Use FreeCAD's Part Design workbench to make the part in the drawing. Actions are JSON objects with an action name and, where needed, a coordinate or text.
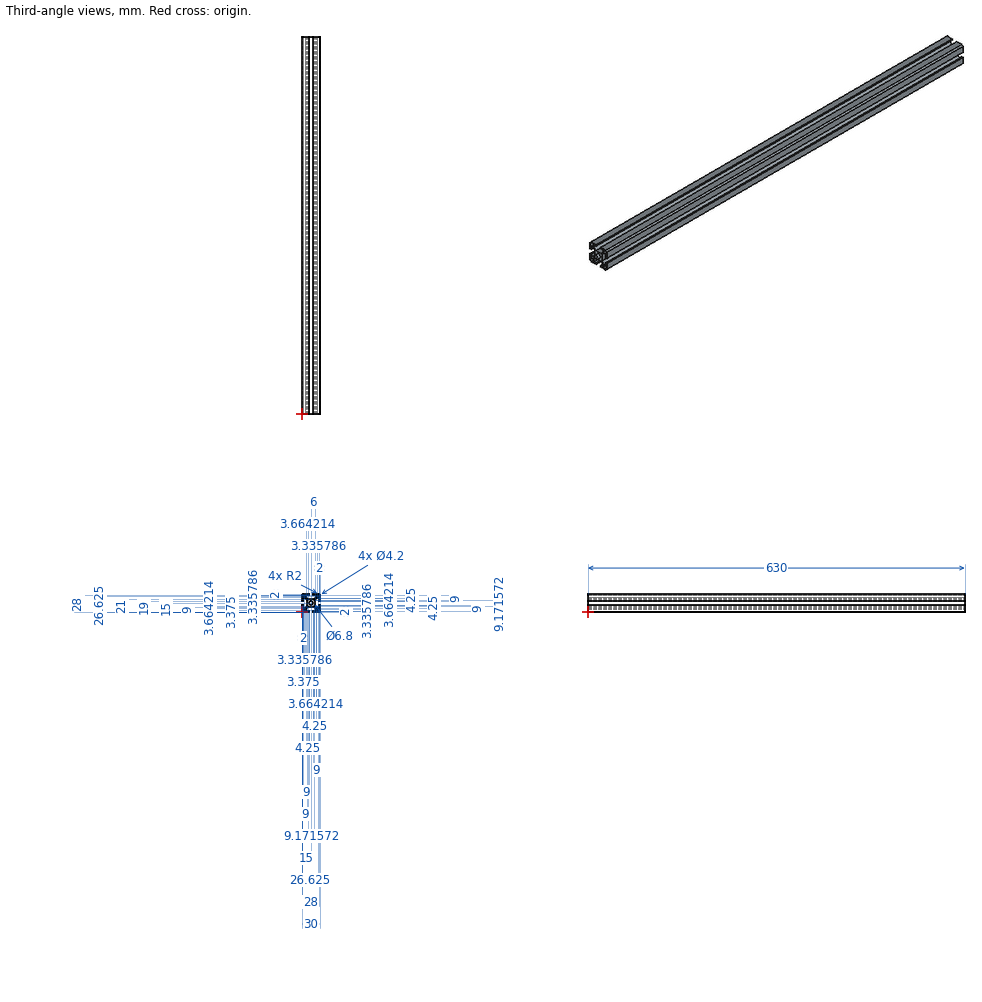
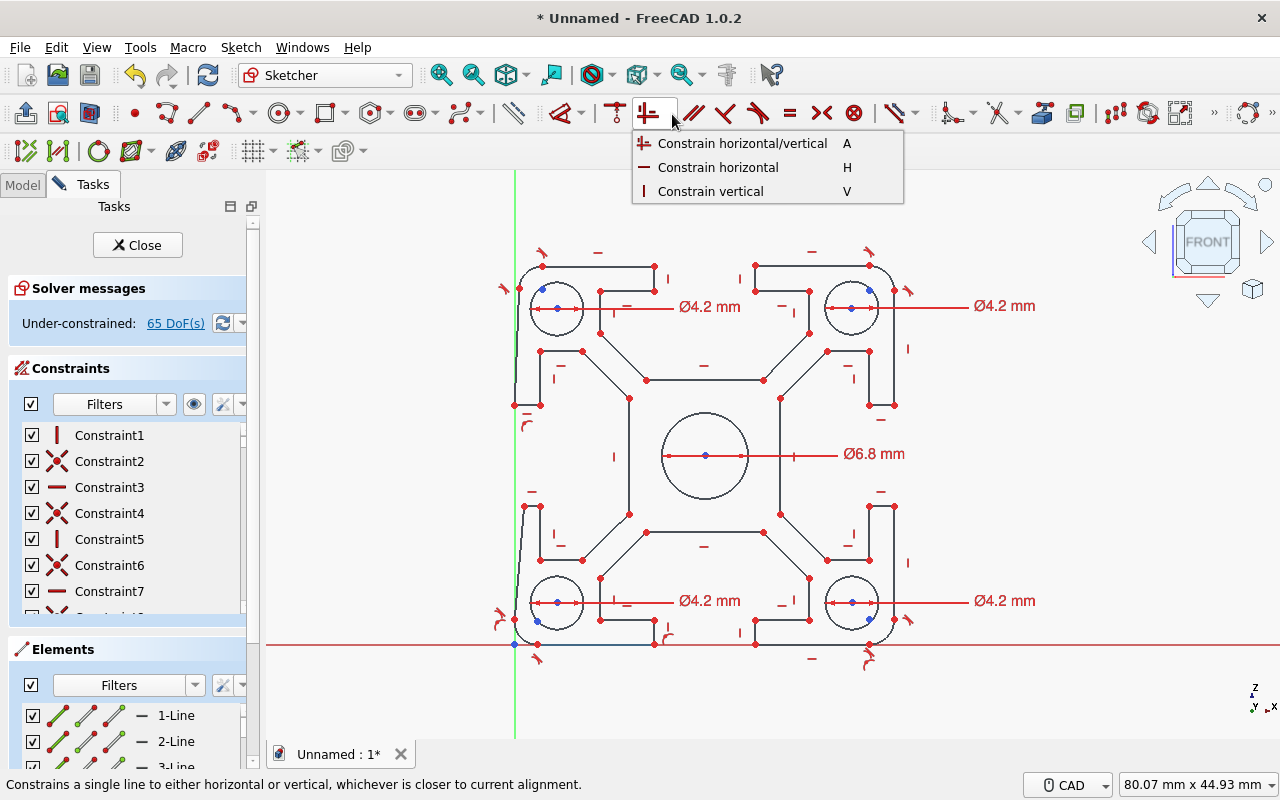
{"action": "left_click", "coordinate": [768, 167]}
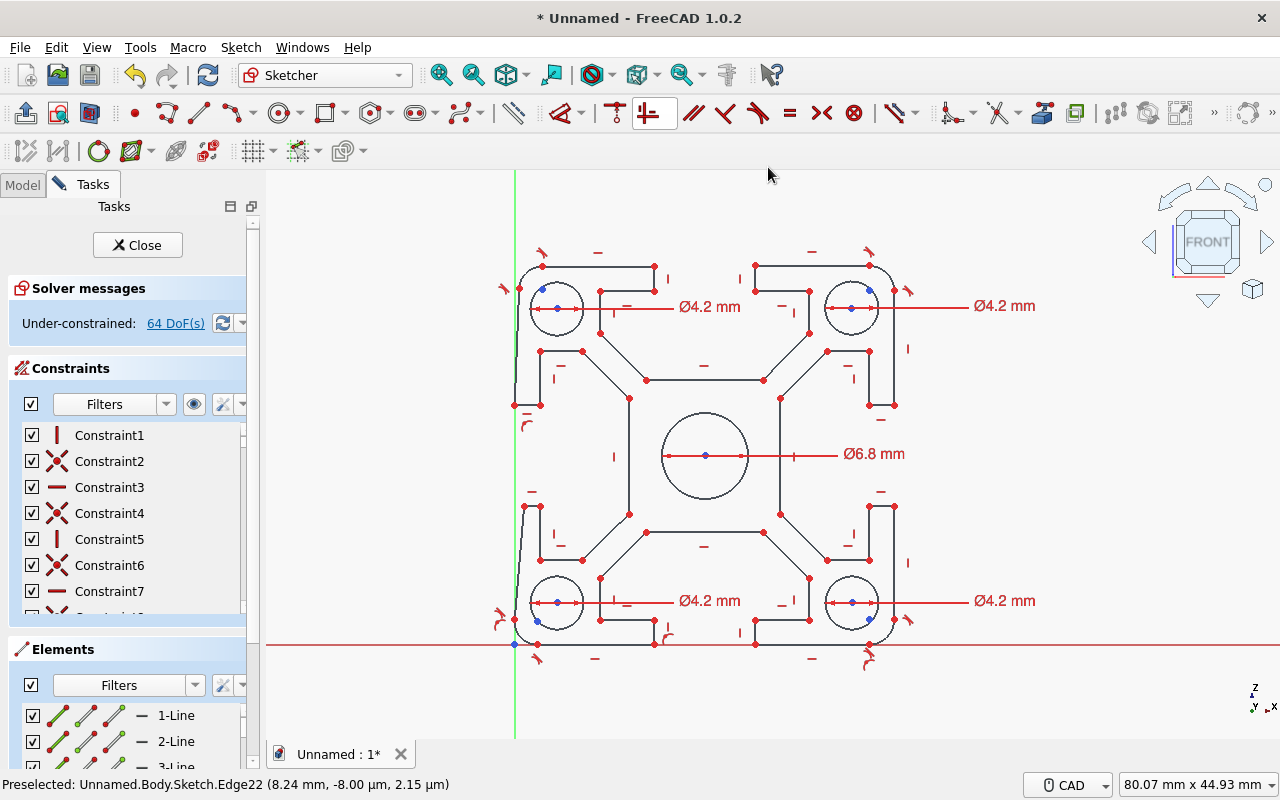
{"action": "left_click", "coordinate": [517, 586]}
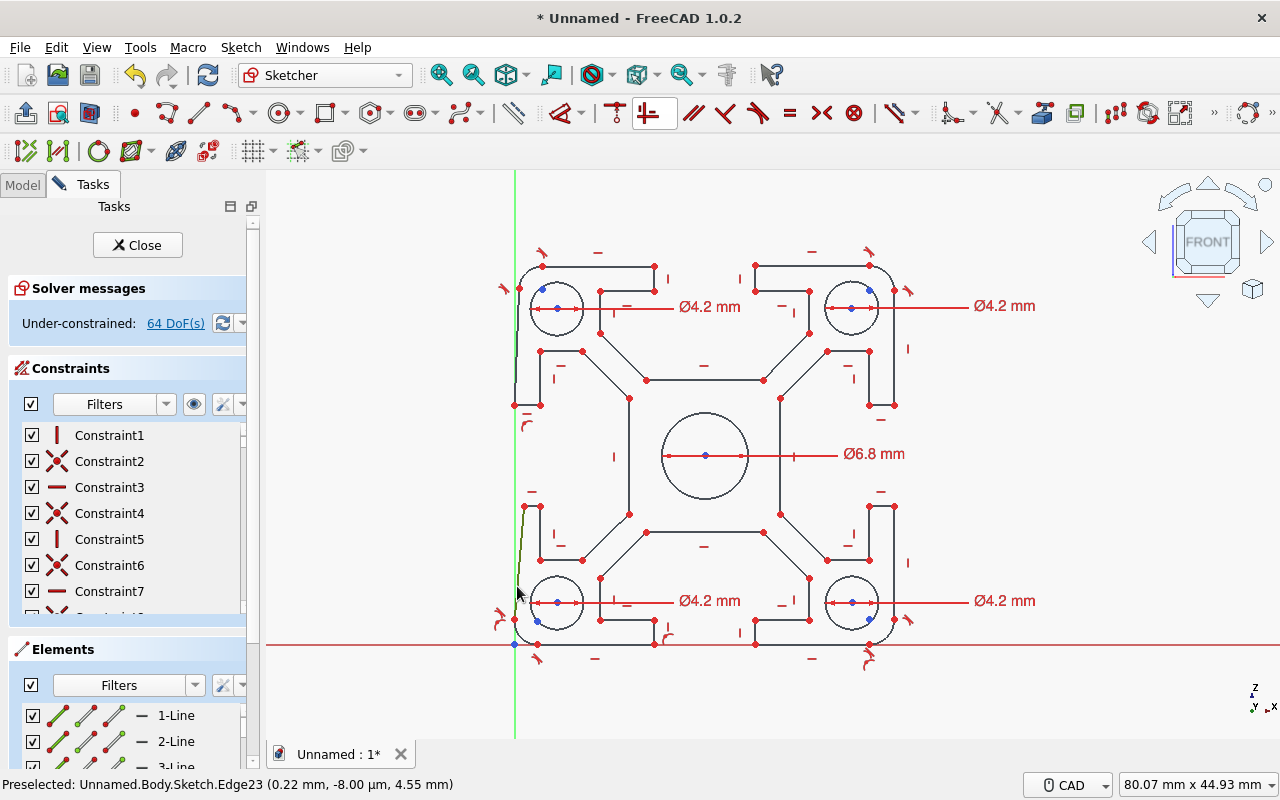
{"action": "left_click", "coordinate": [672, 114]}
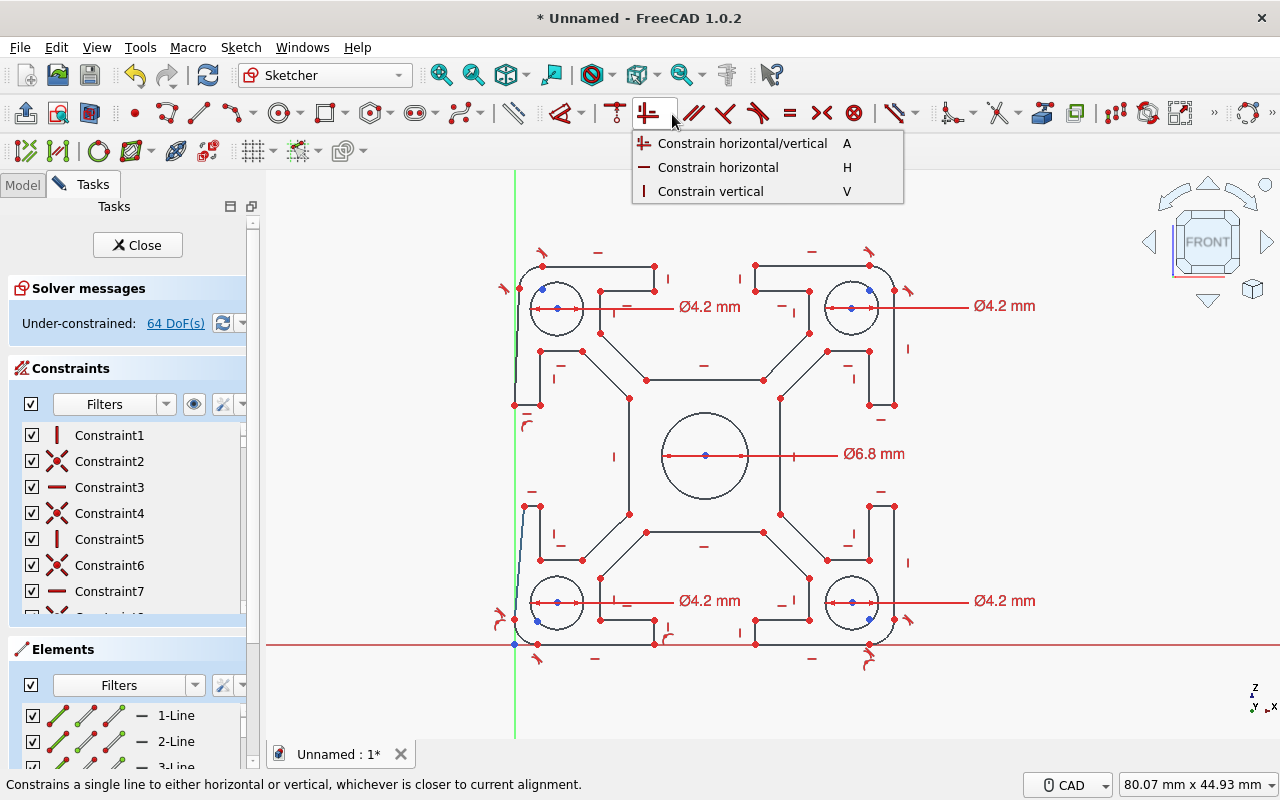
{"action": "left_click", "coordinate": [768, 191]}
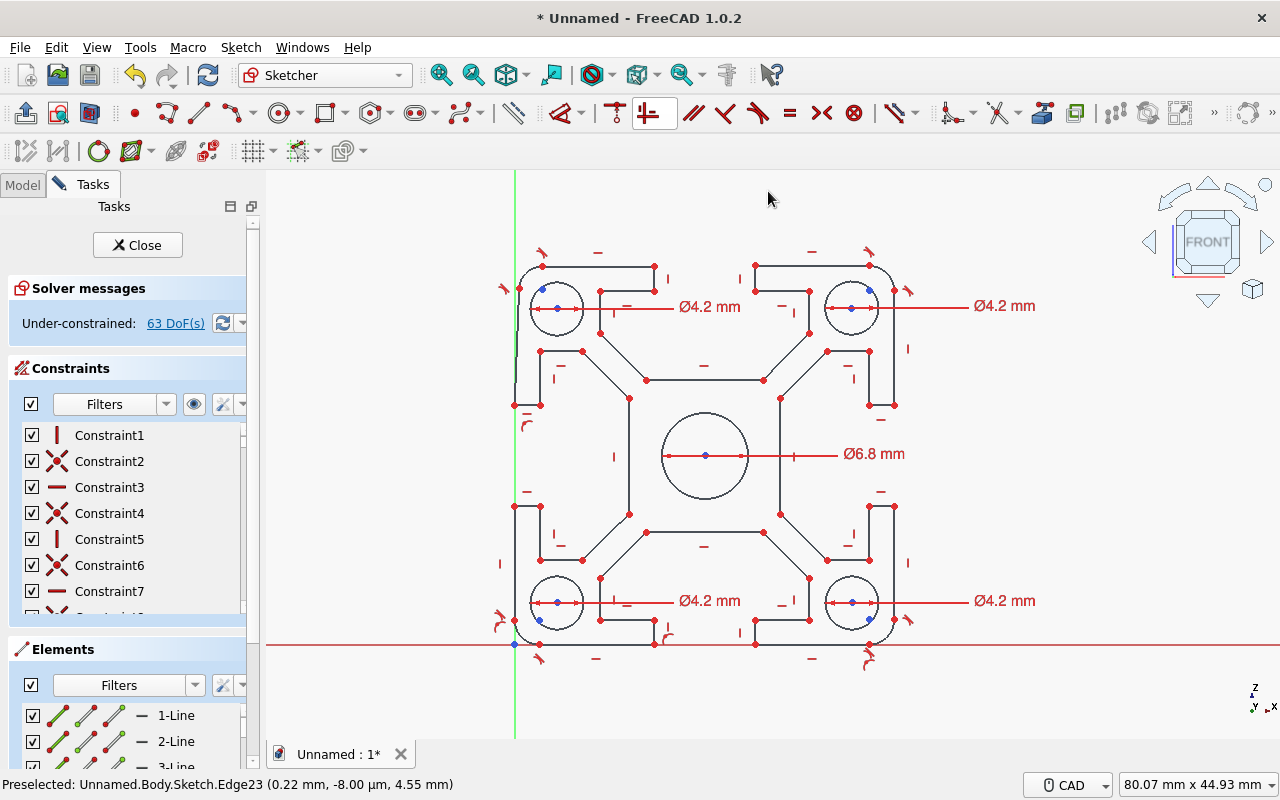
{"action": "left_click", "coordinate": [516, 370]}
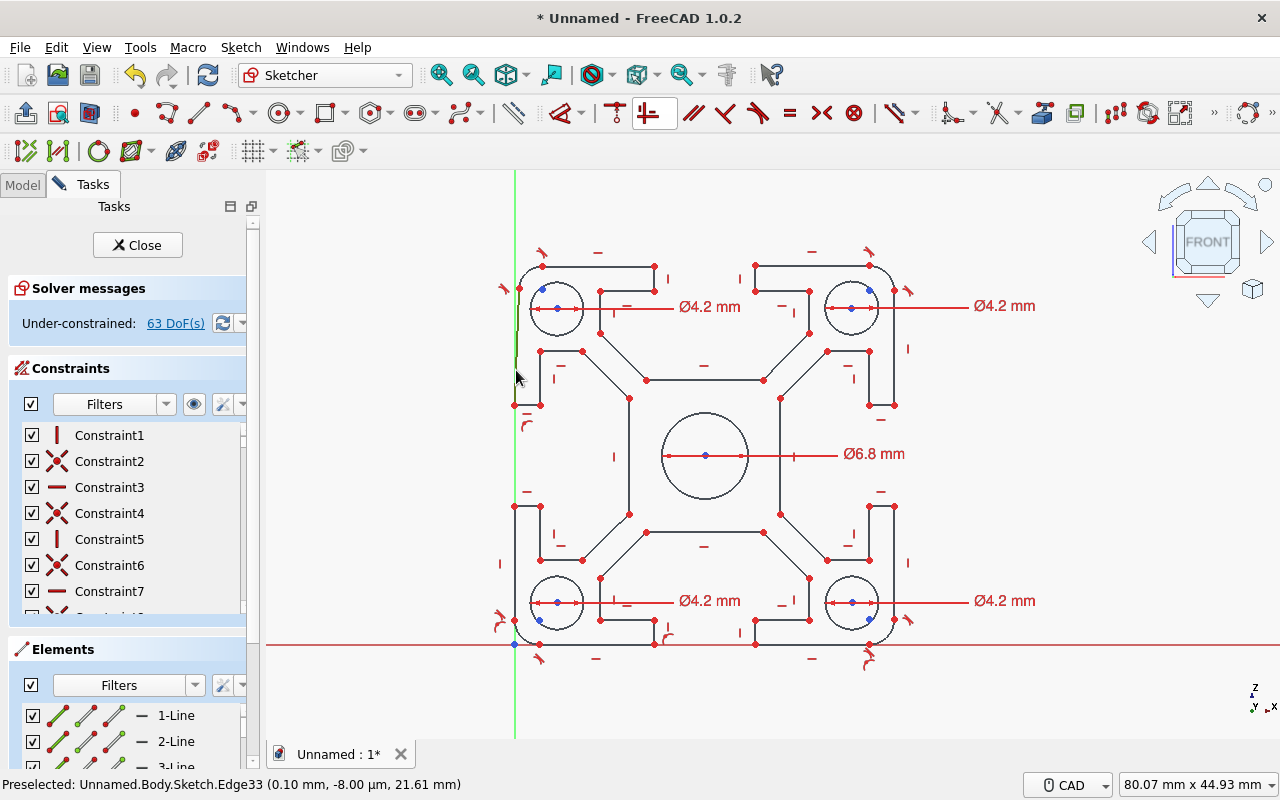
{"action": "left_click", "coordinate": [672, 114]}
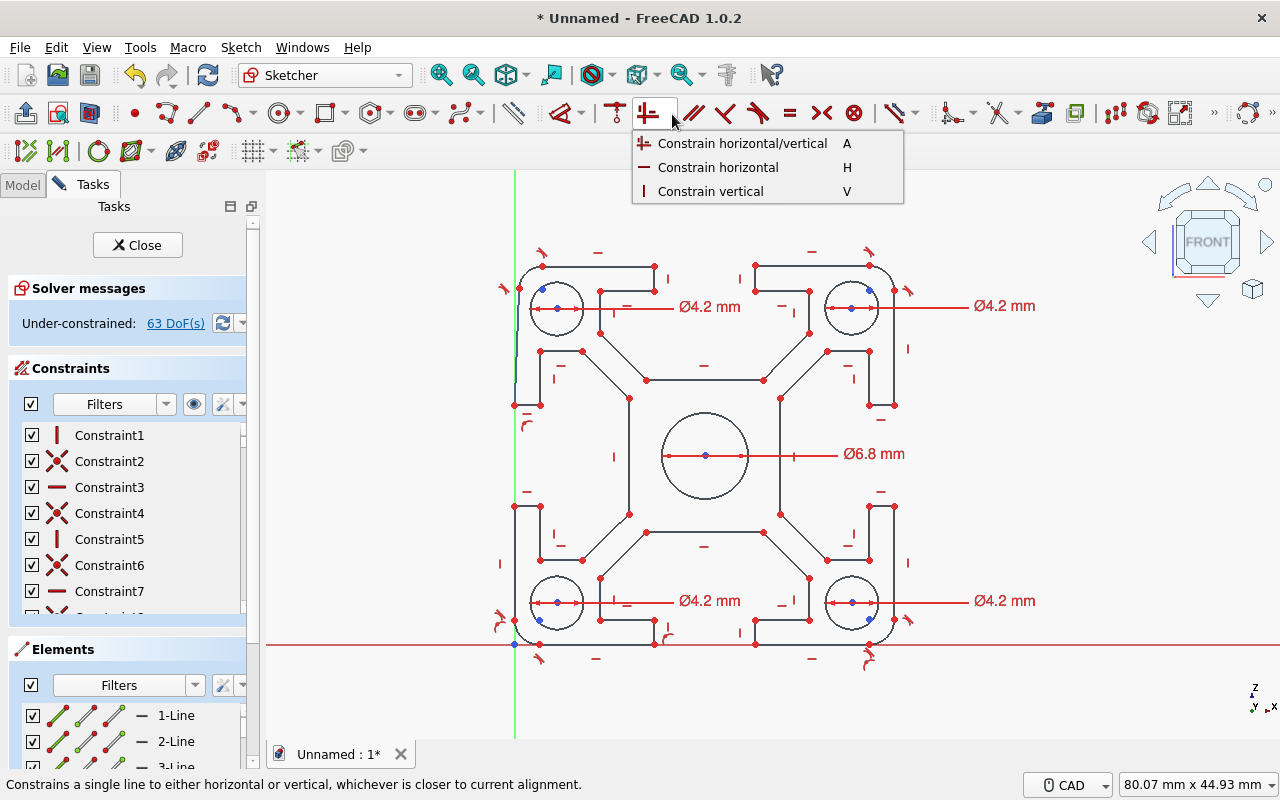
{"action": "left_click", "coordinate": [768, 191]}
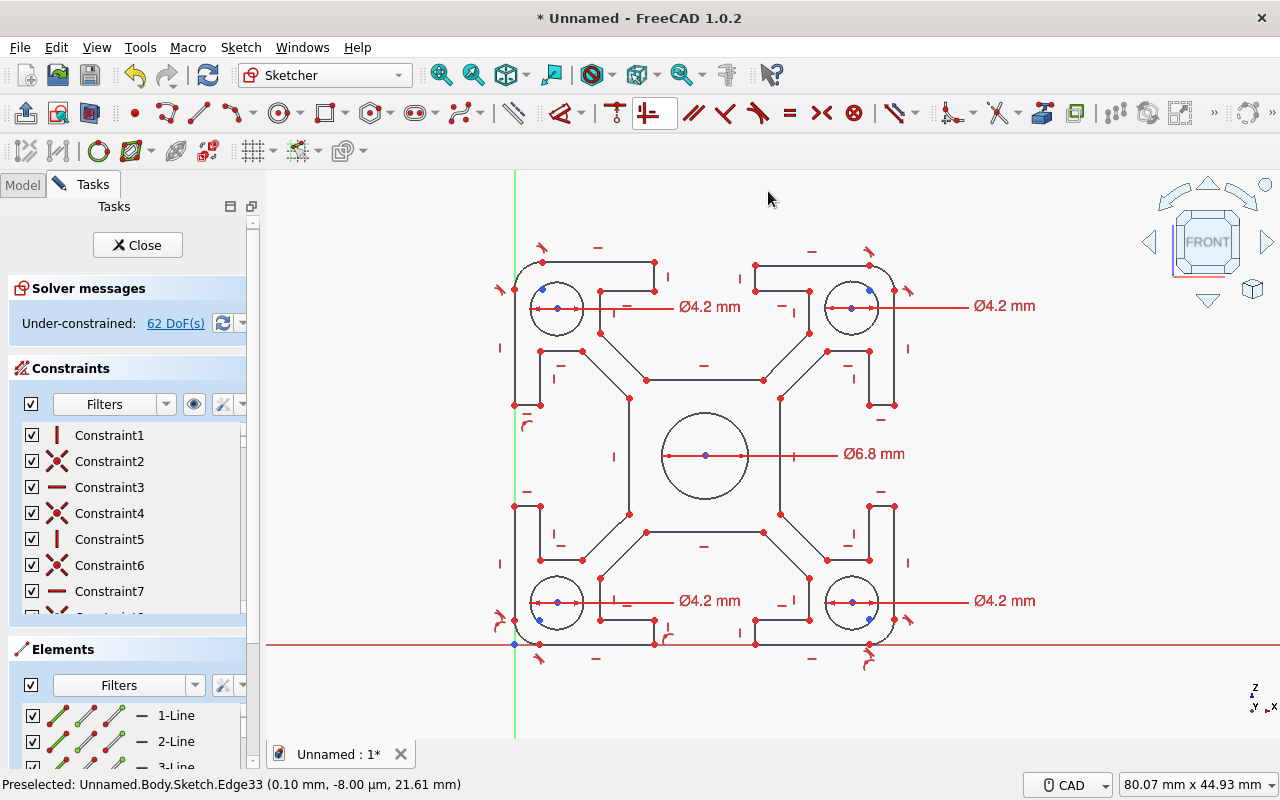
{"action": "left_click", "coordinate": [880, 642]}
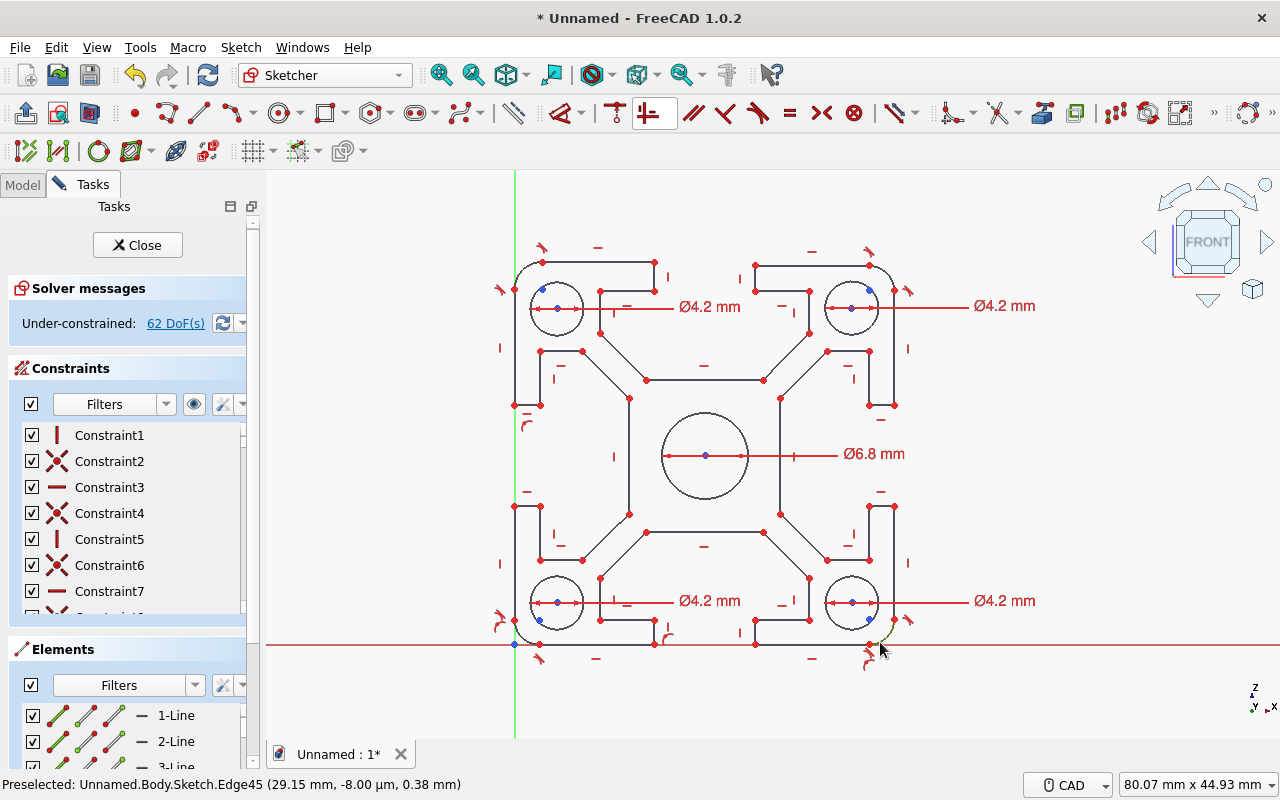
{"action": "left_click", "coordinate": [517, 631]}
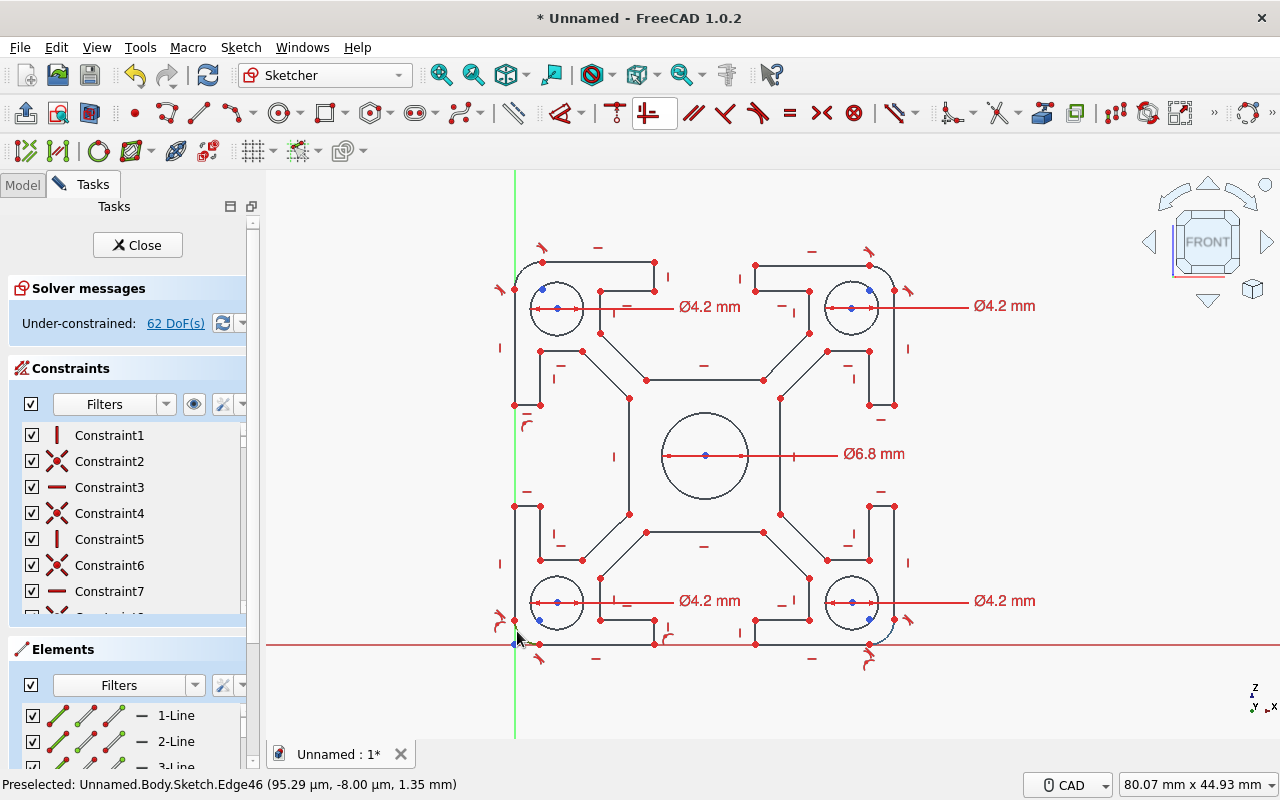
{"action": "left_click", "coordinate": [530, 265]}